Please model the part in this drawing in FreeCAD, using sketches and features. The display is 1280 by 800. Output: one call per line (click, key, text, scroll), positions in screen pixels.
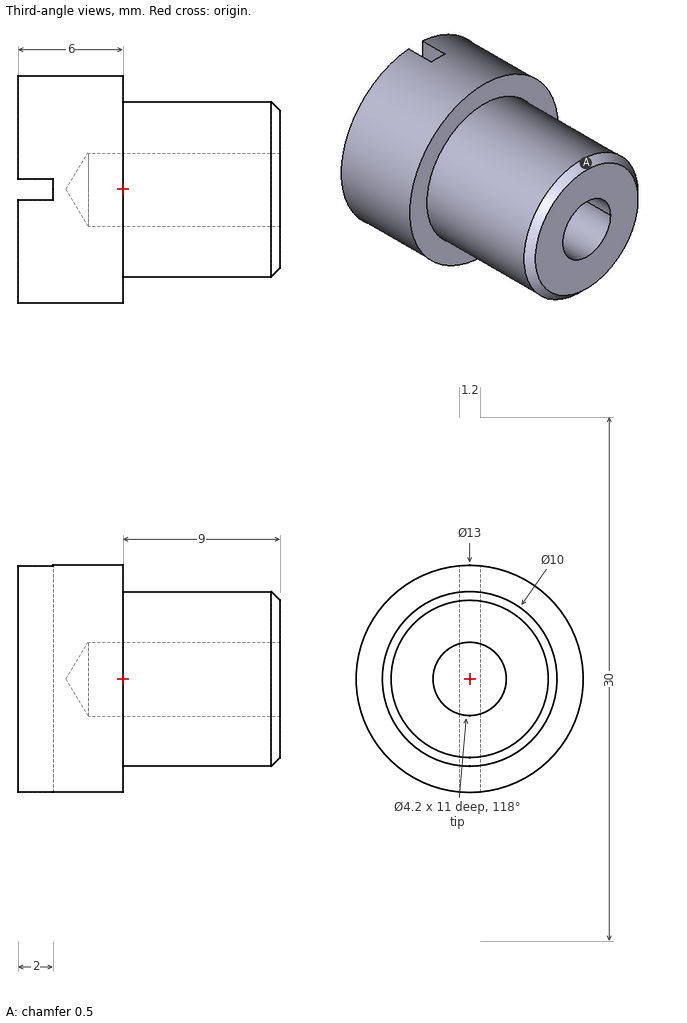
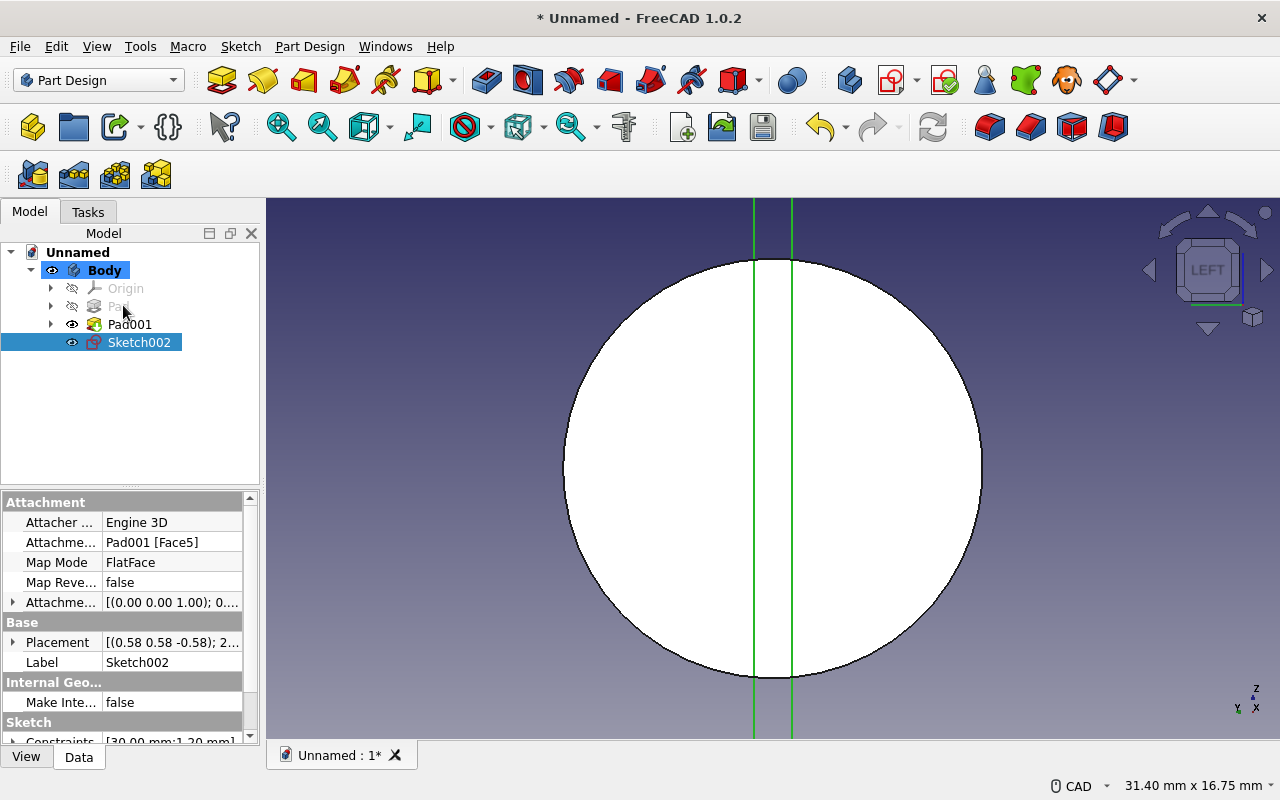
click(487, 80)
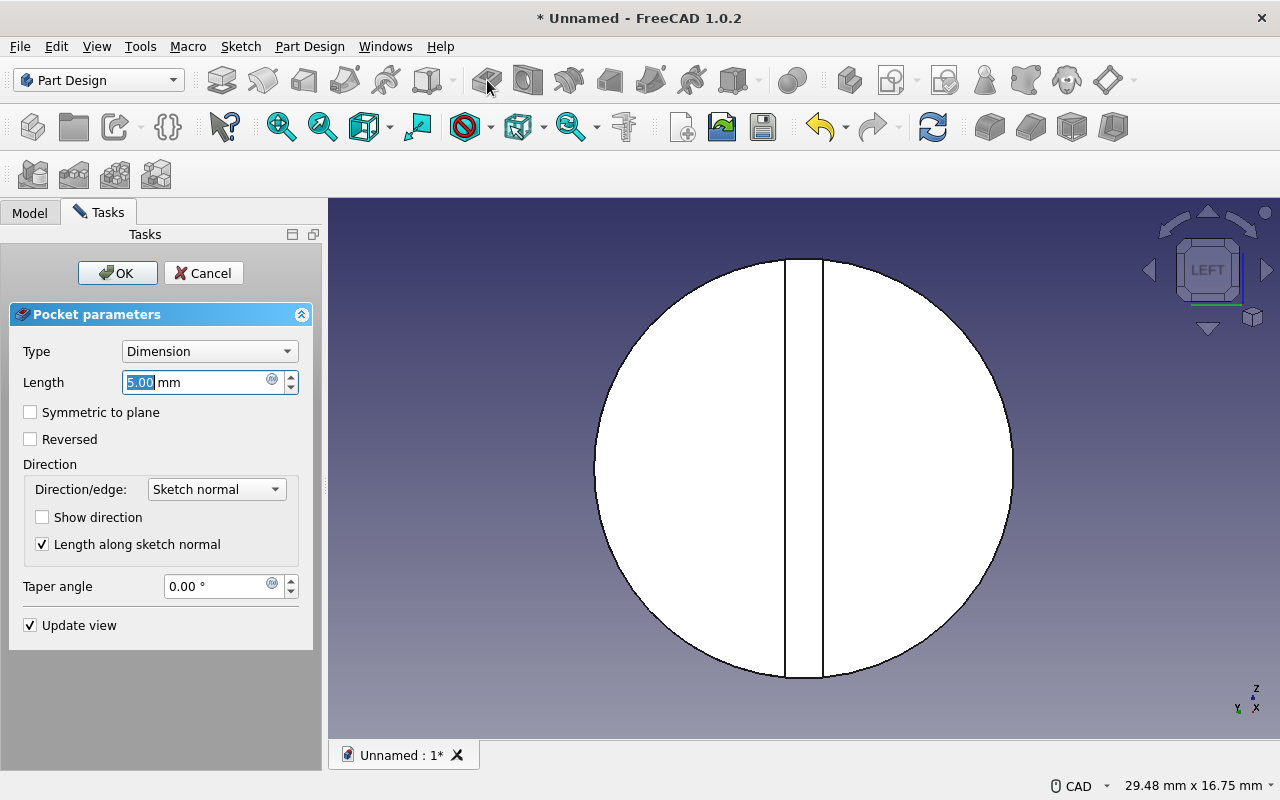
text(2)
key(Tab)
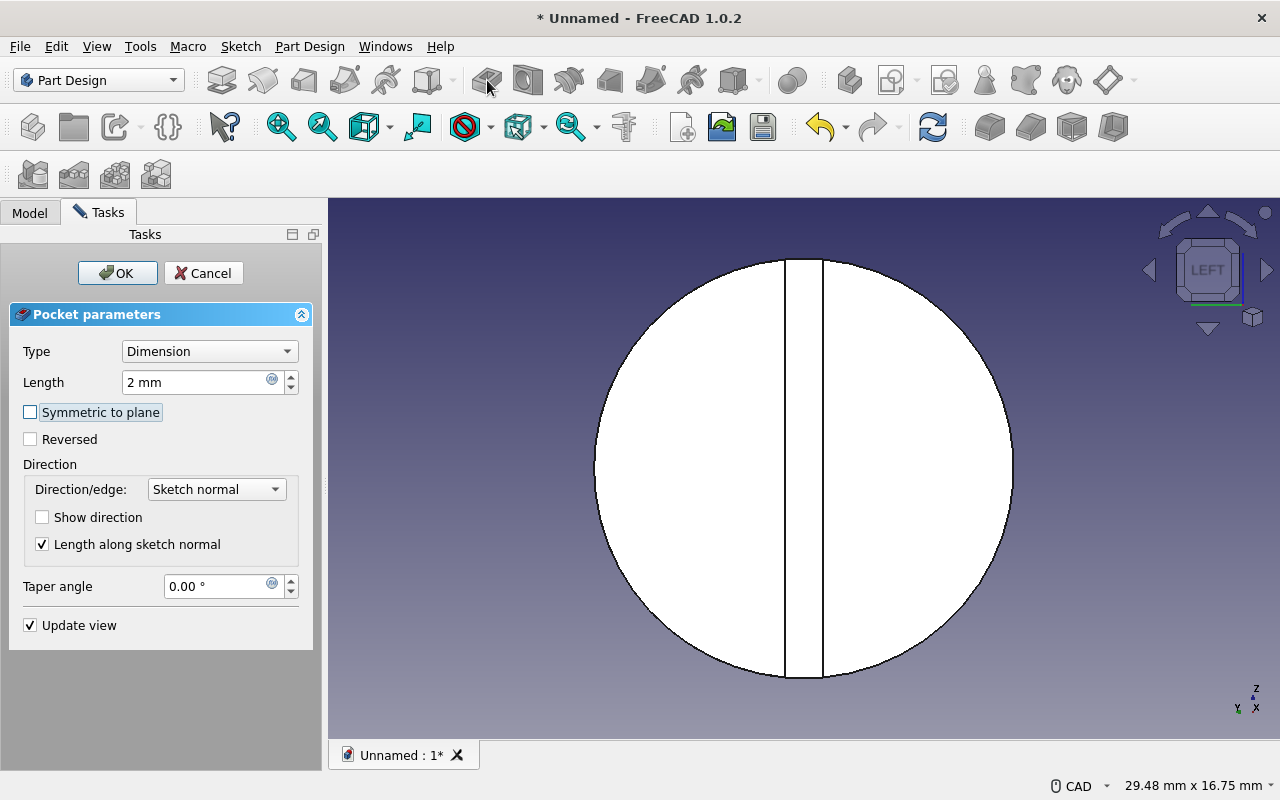
click(118, 273)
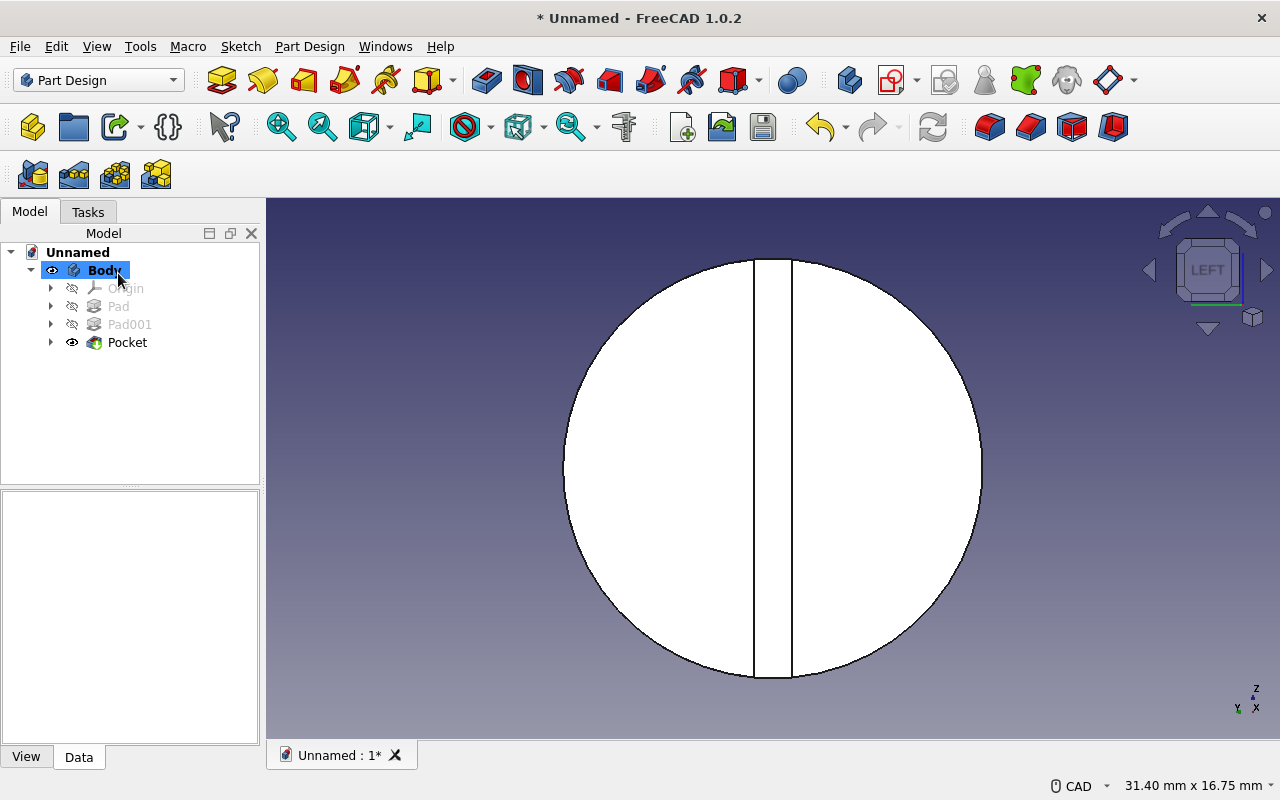
key(0)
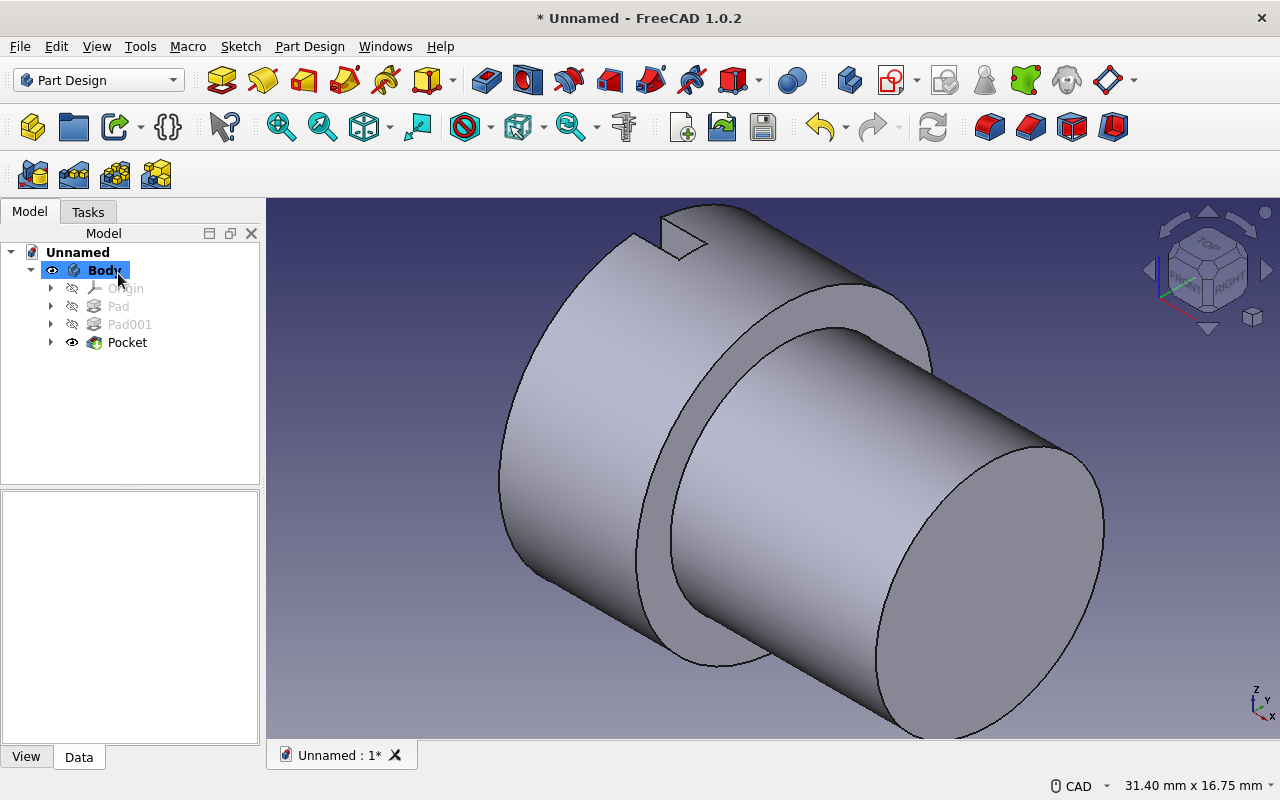
click(282, 128)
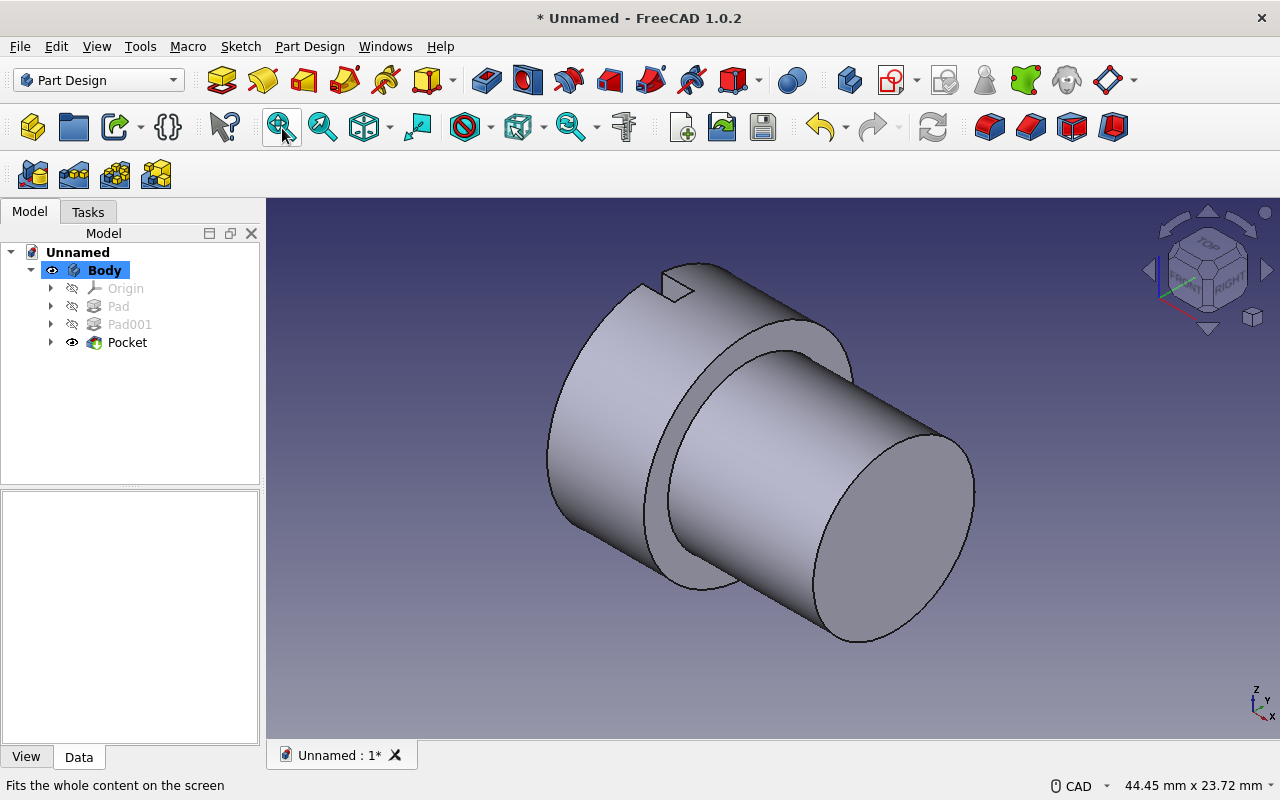
click(894, 537)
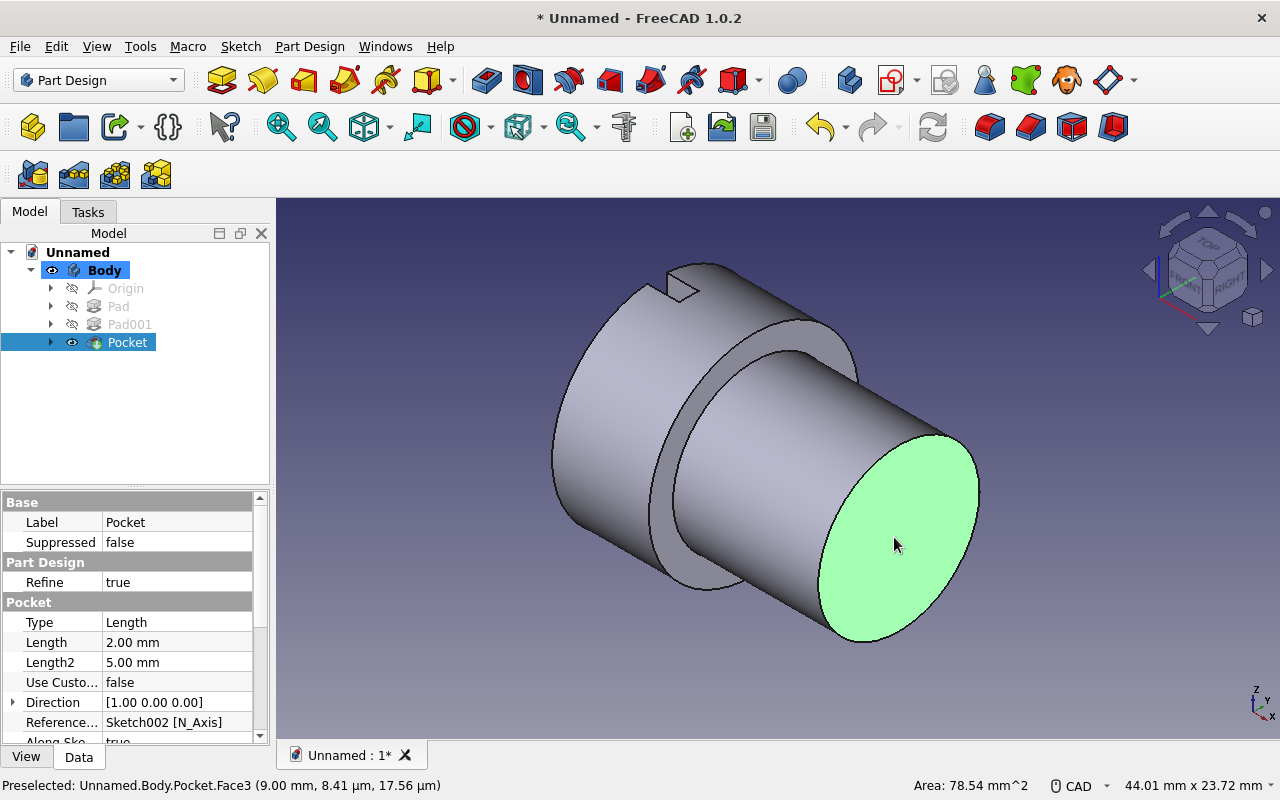
click(890, 80)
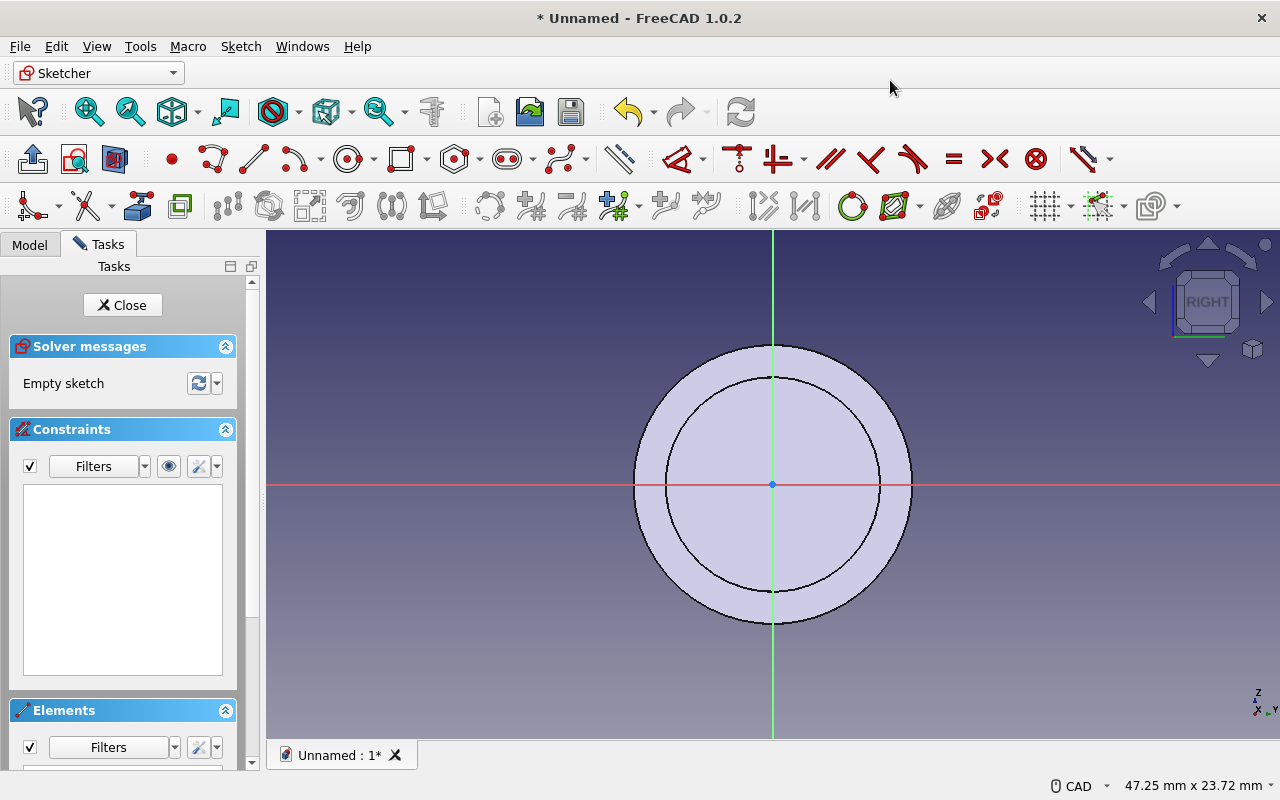
scroll(802, 484, up, 6)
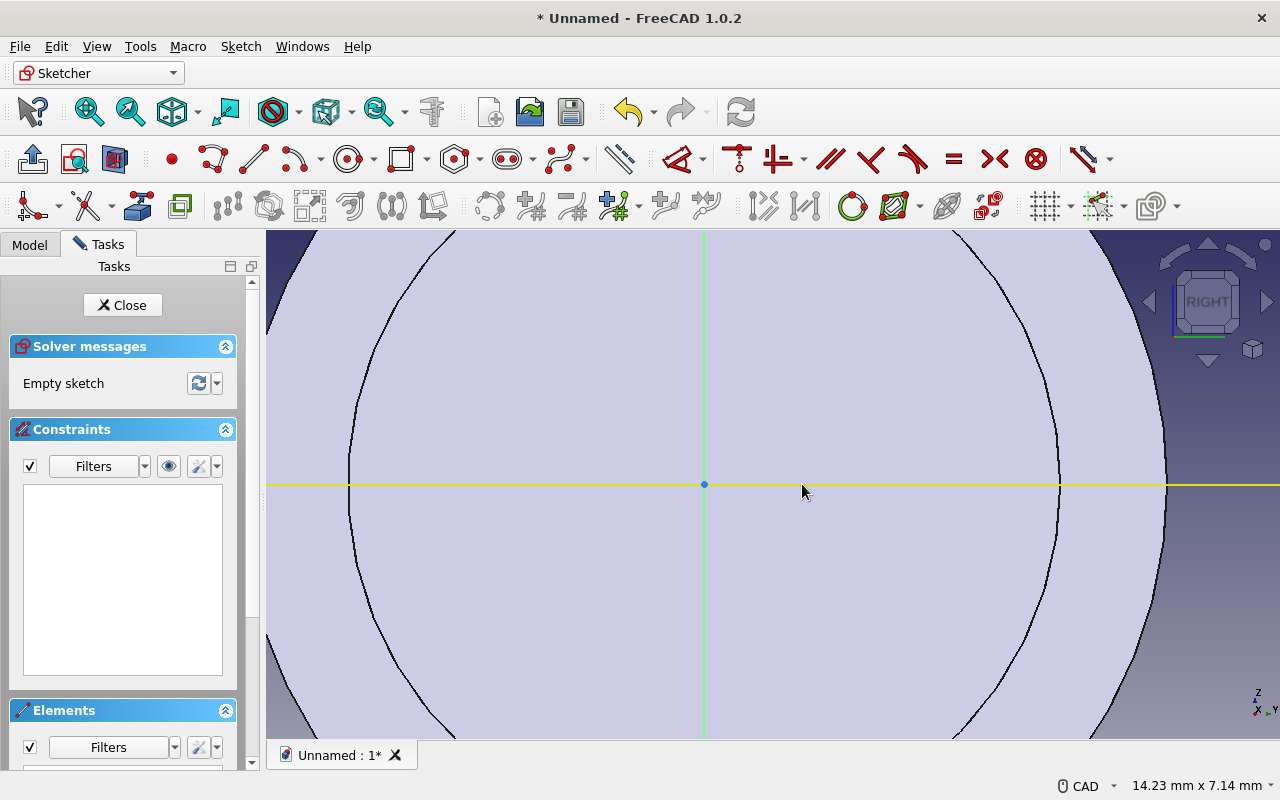
click(348, 160)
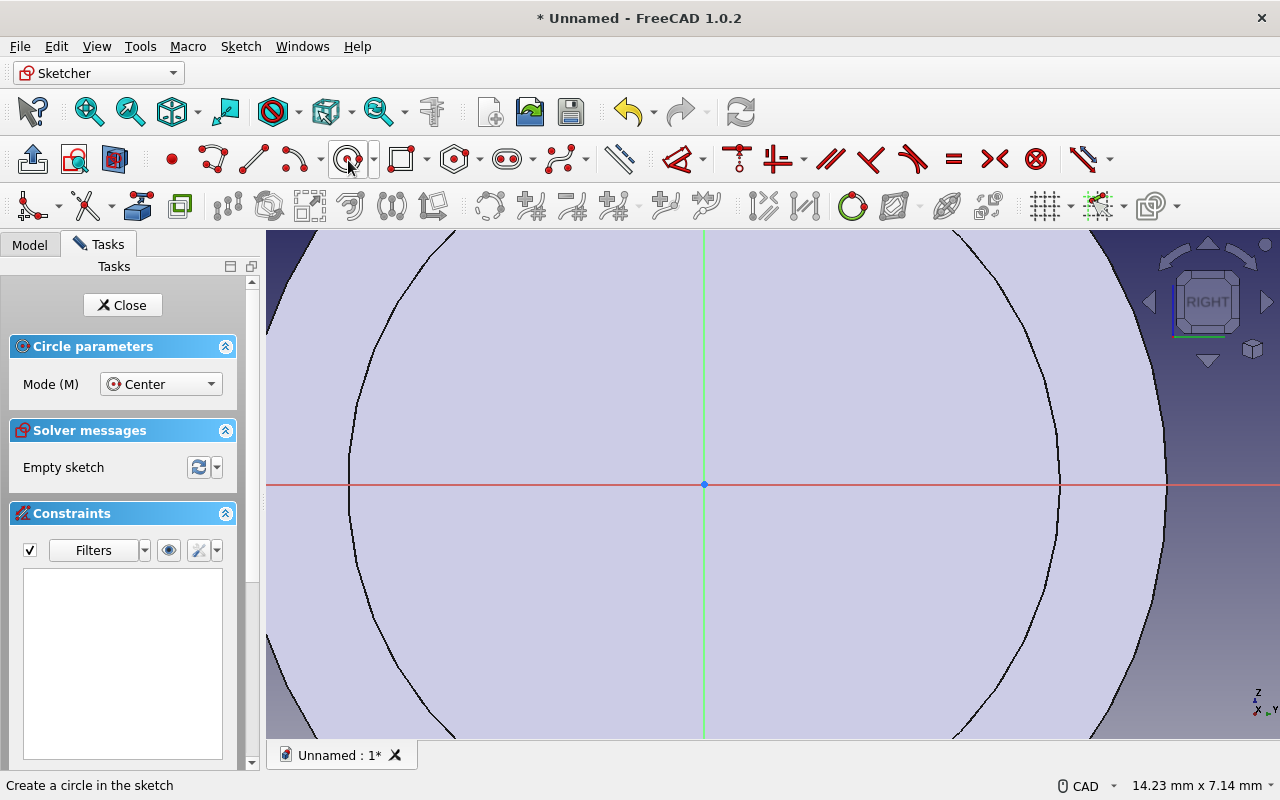
click(704, 484)
move(810, 379)